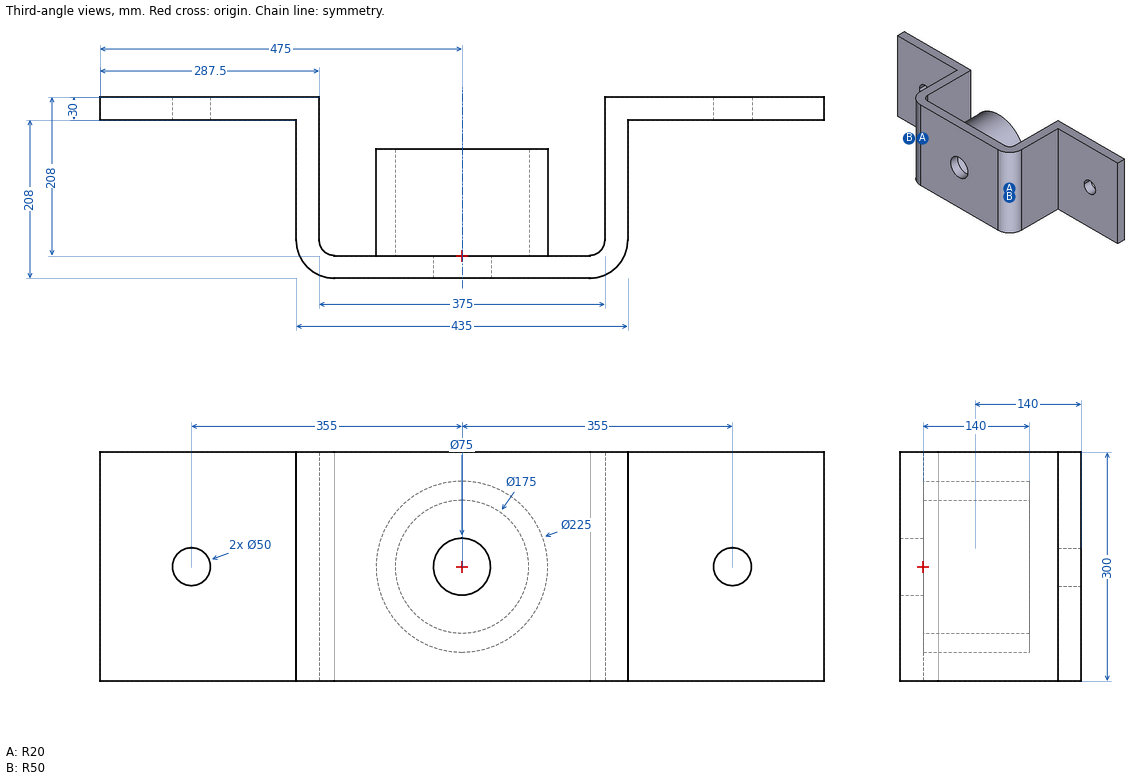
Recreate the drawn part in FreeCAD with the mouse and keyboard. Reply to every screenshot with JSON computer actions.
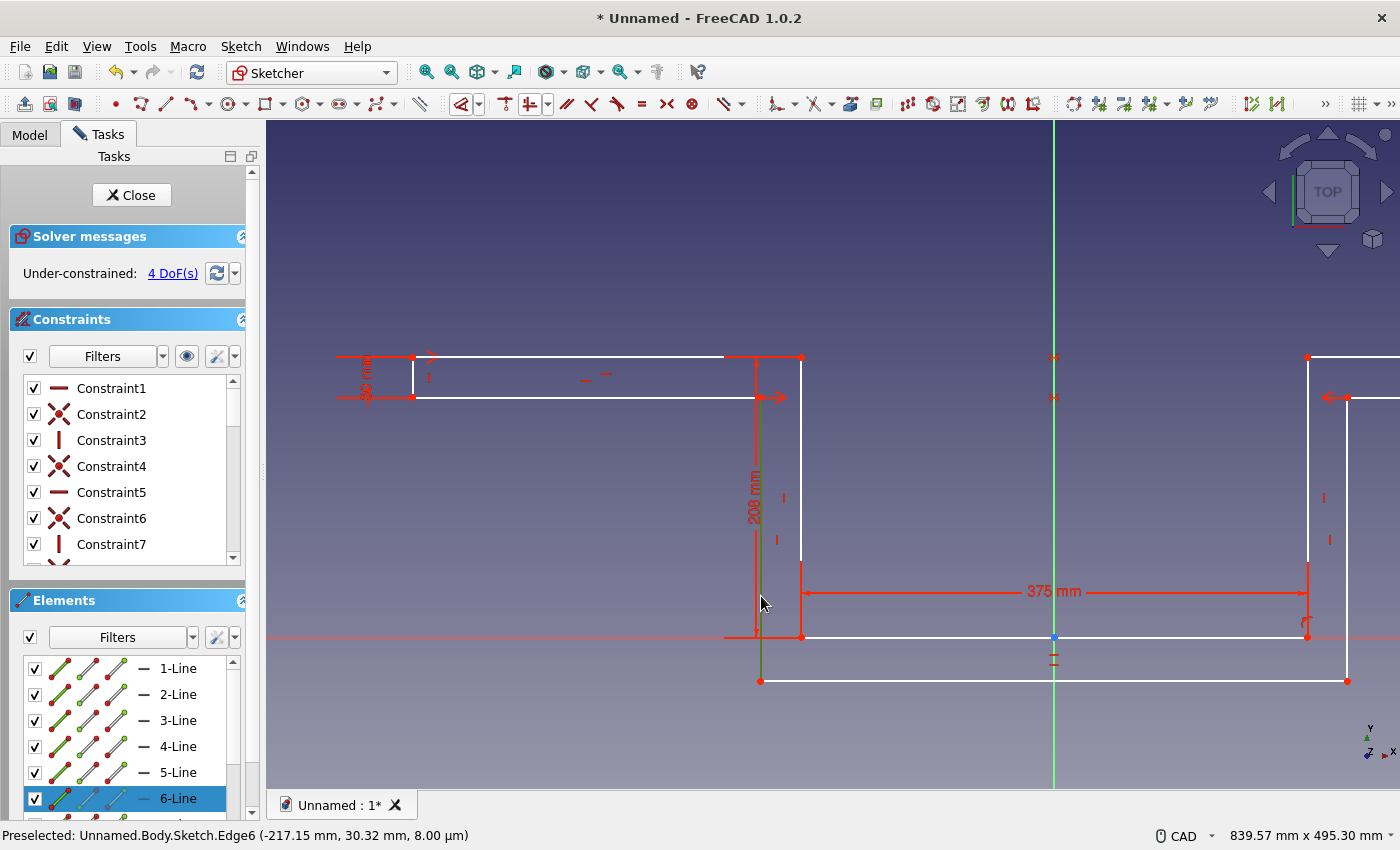
{"action": "left_click", "coordinate": [478, 104]}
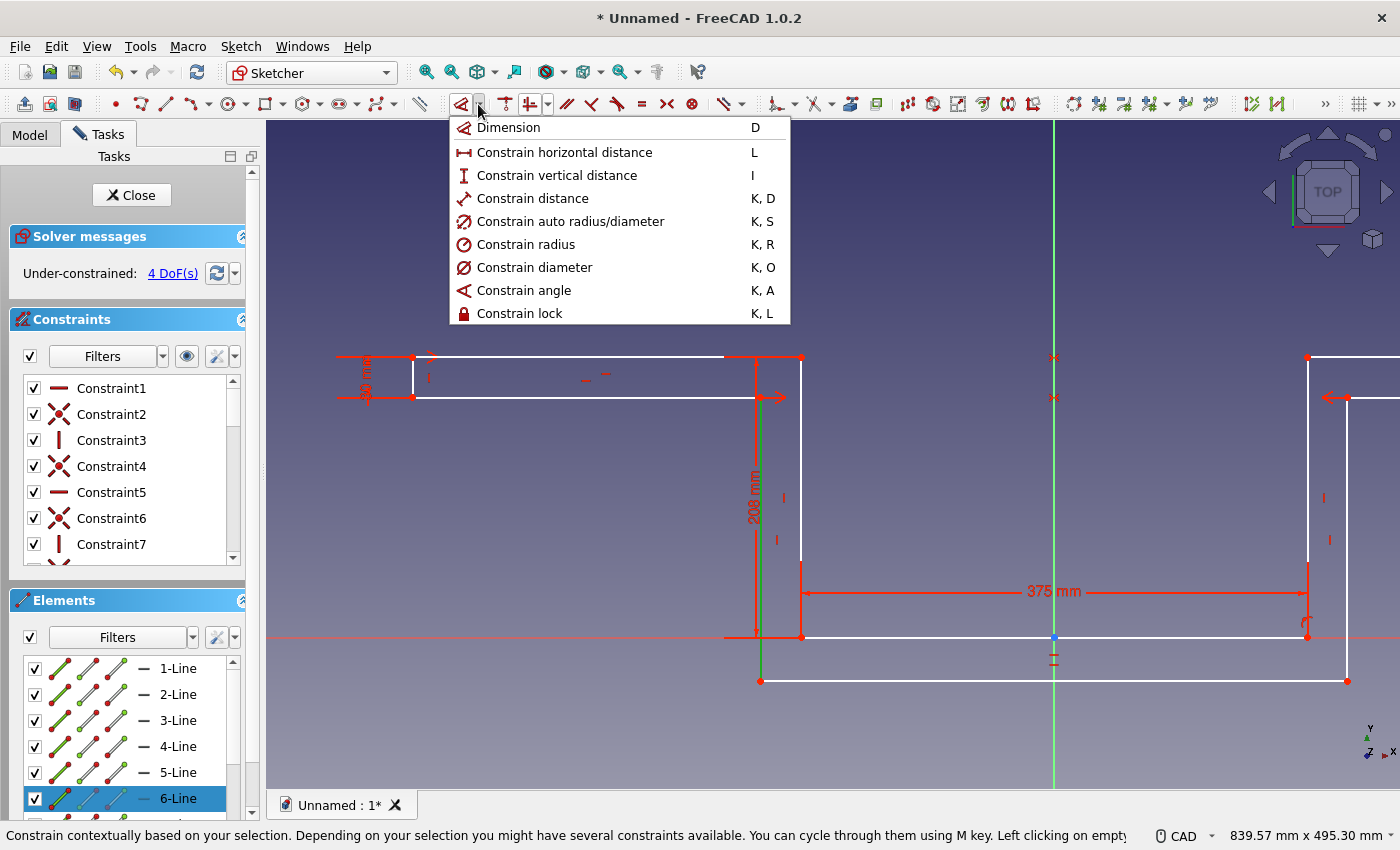
{"action": "left_click", "coordinate": [620, 176]}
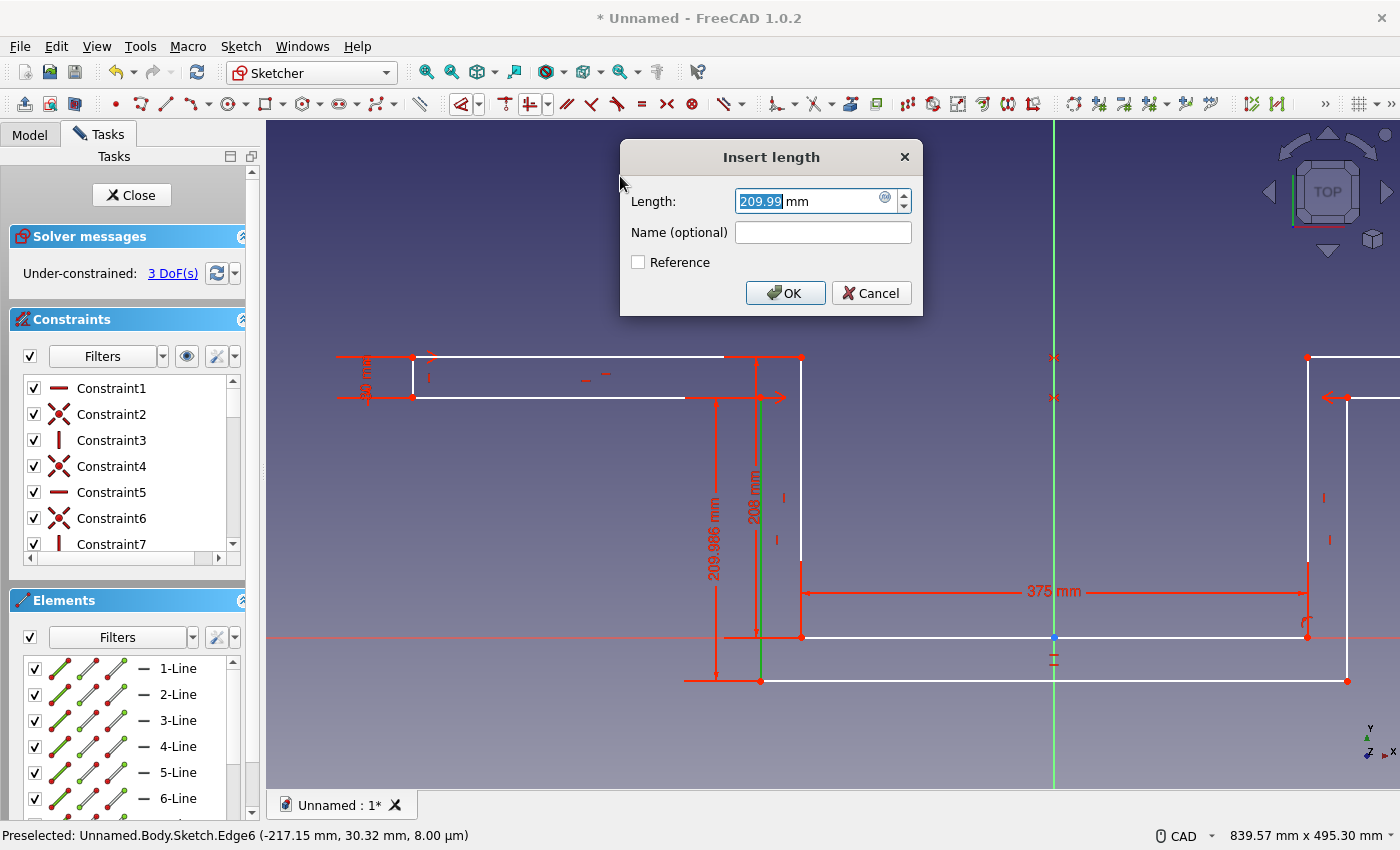
{"action": "type", "text": "208"}
{"action": "key", "text": "Return"}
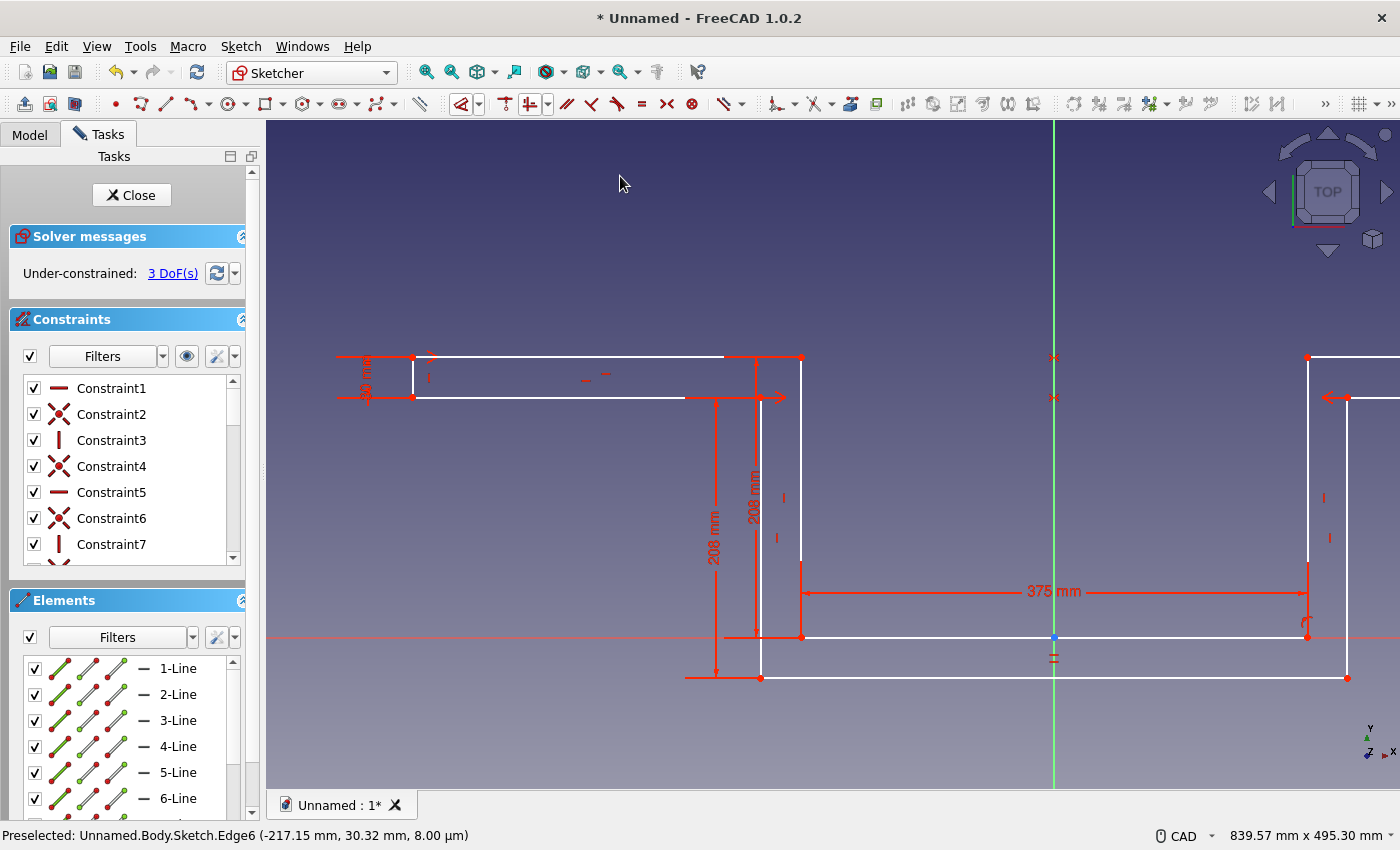
{"action": "left_click", "coordinate": [937, 678]}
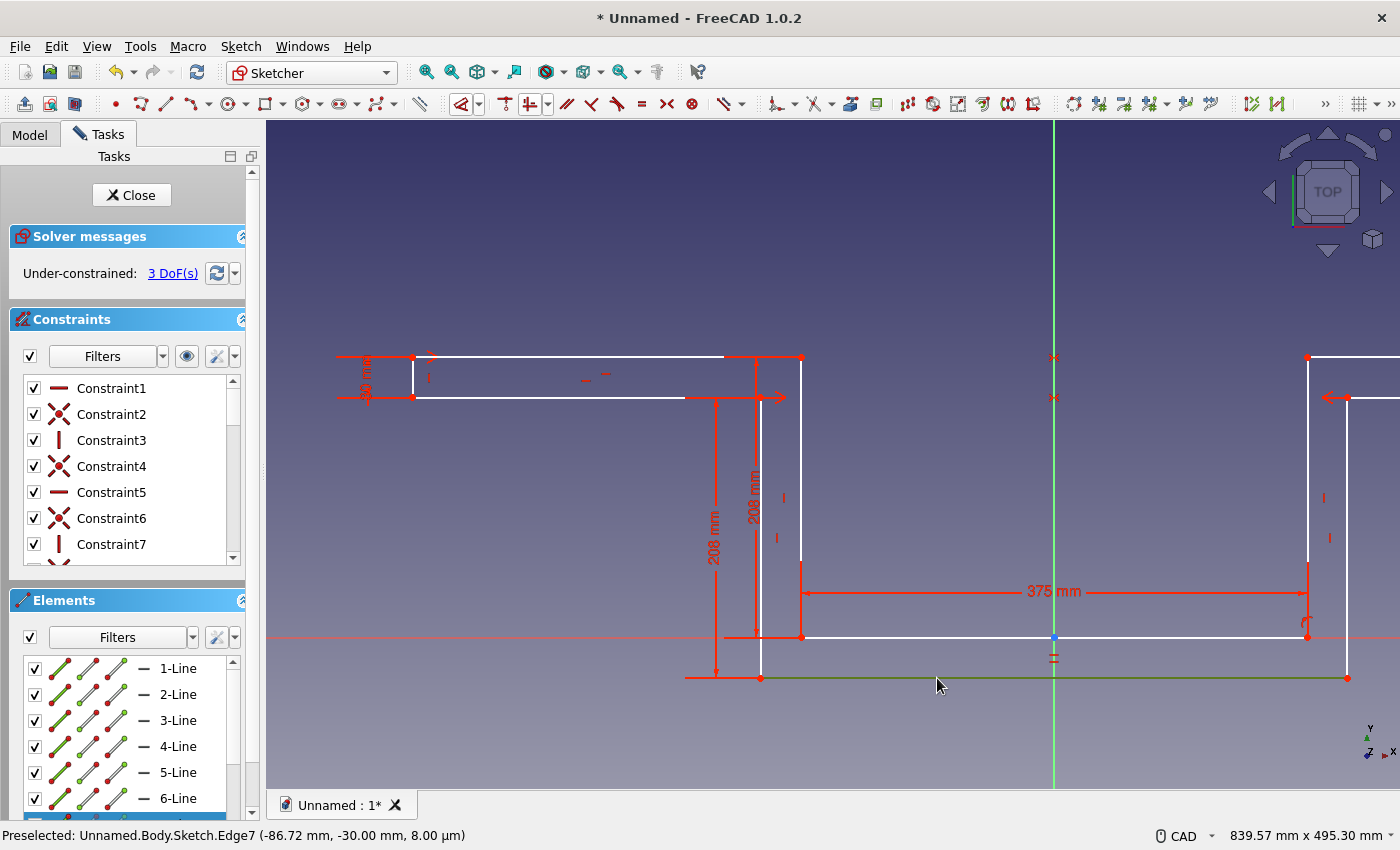
{"action": "key", "text": "l"}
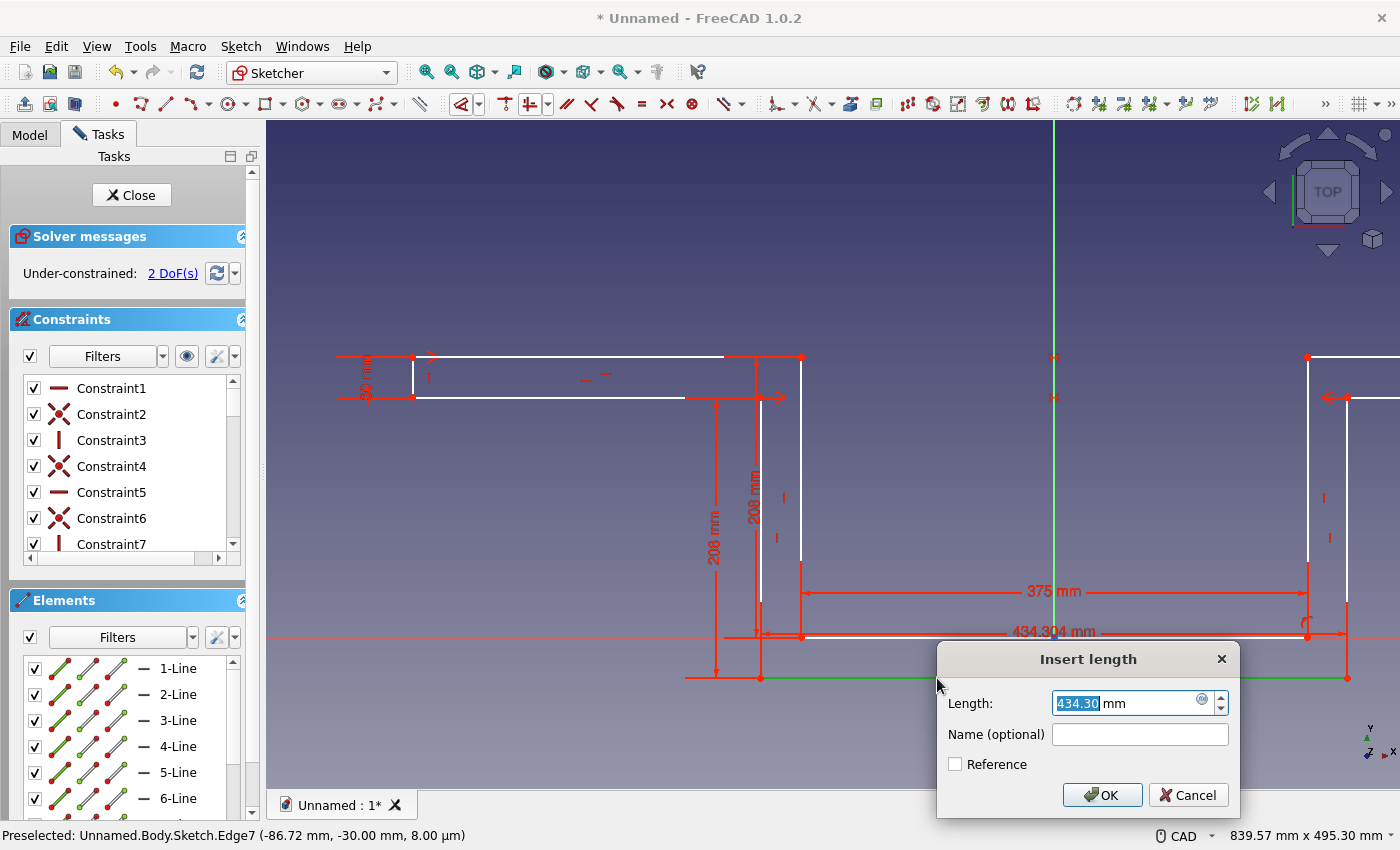
{"action": "type", "text": "435"}
{"action": "key", "text": "Return"}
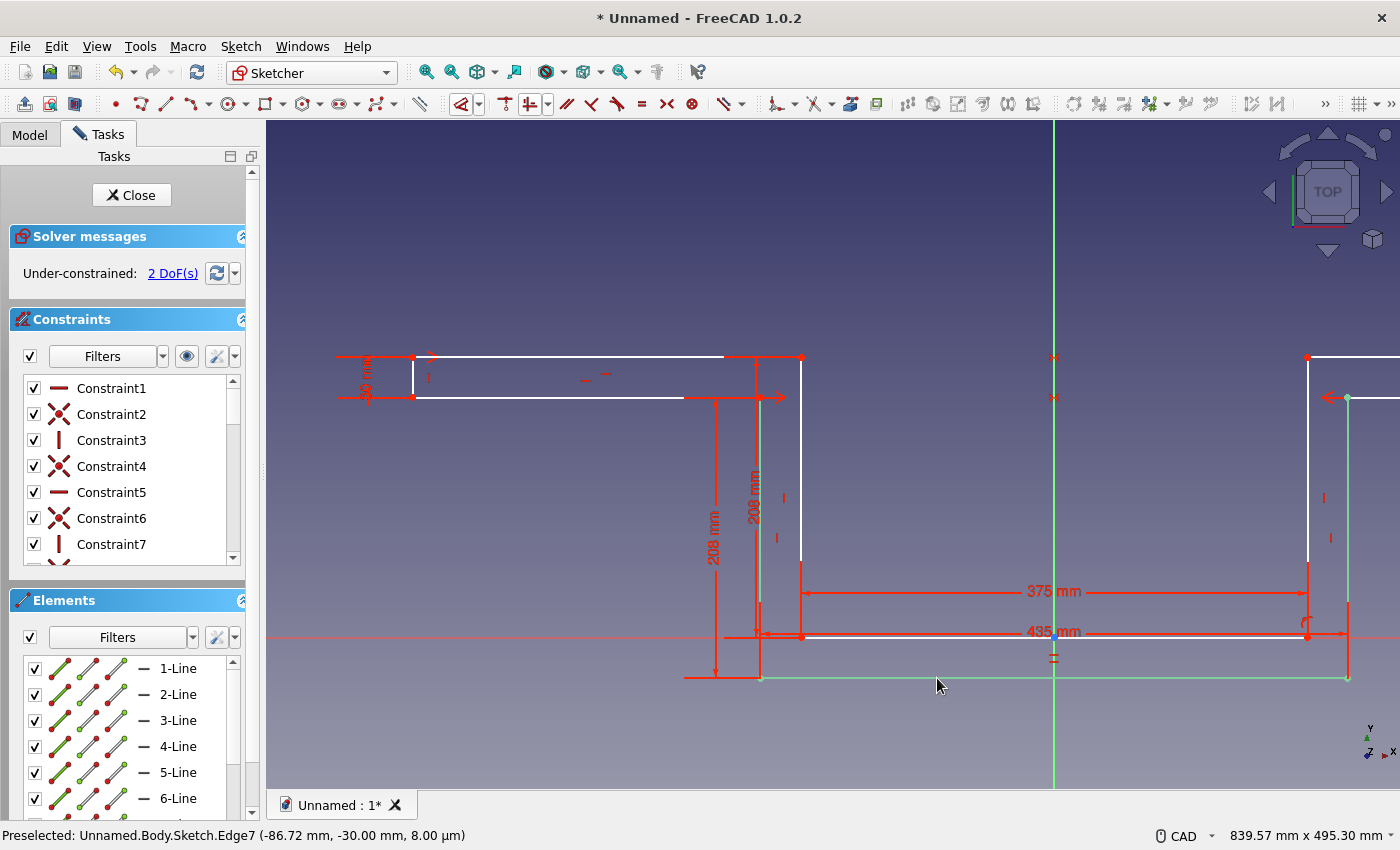
{"action": "left_click", "coordinate": [413, 357]}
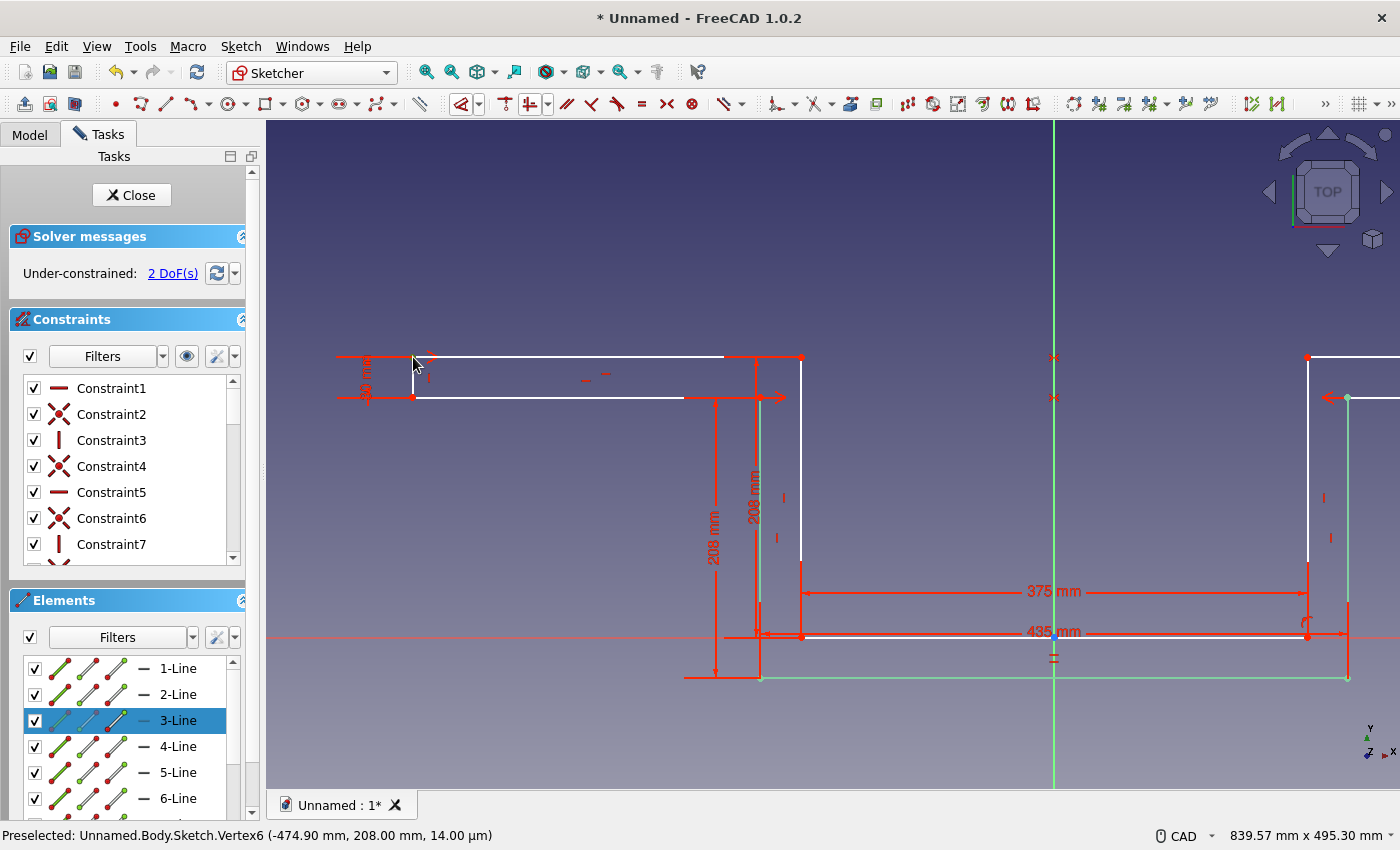
{"action": "key", "text": "l"}